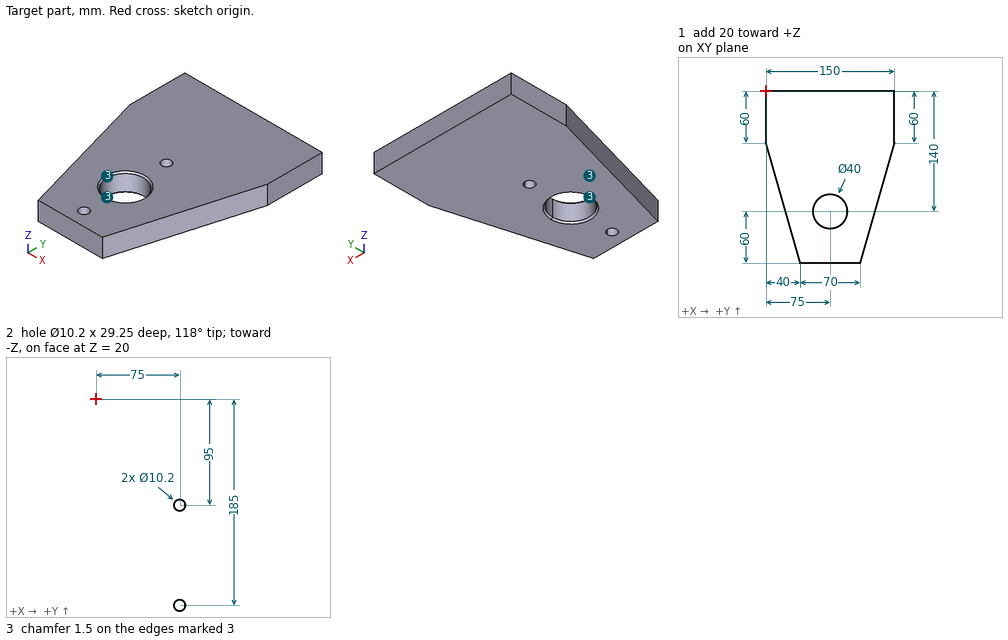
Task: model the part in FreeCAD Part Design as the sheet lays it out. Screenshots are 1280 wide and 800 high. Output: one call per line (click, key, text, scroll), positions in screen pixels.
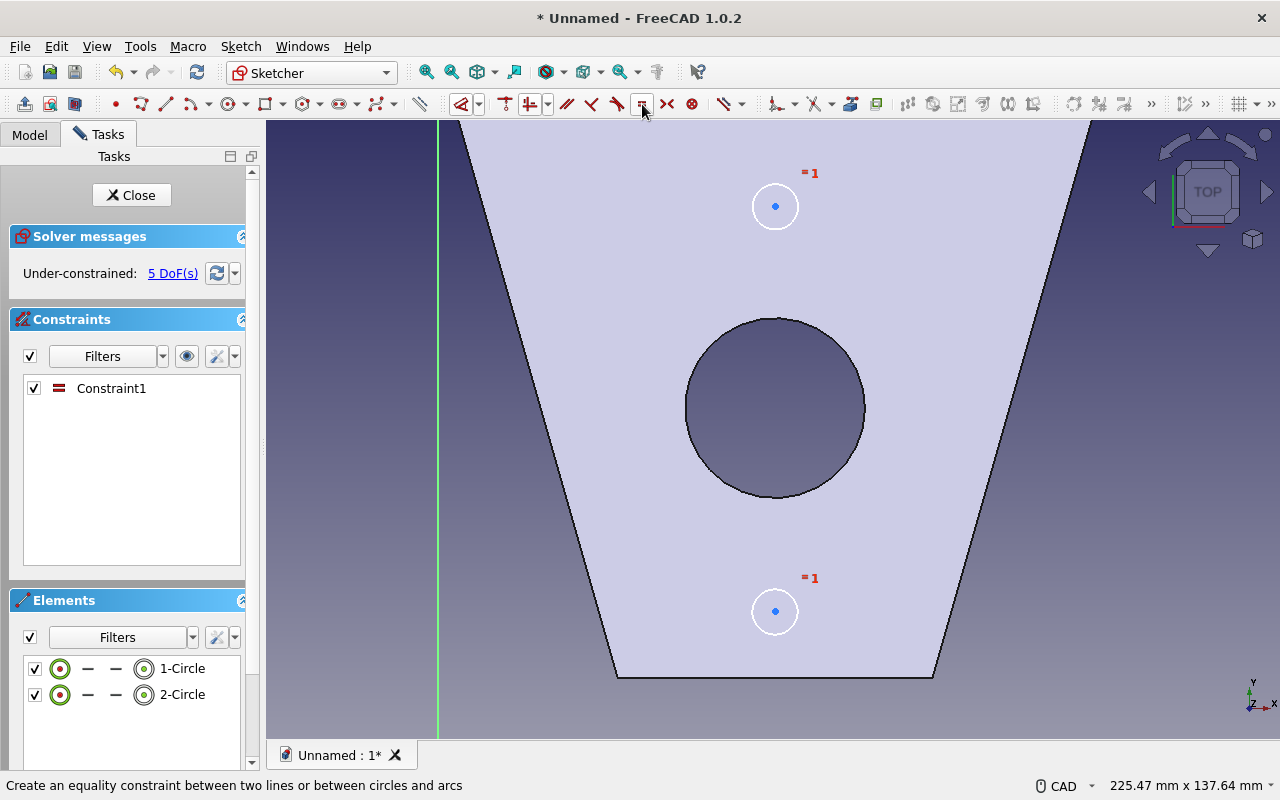
click(775, 207)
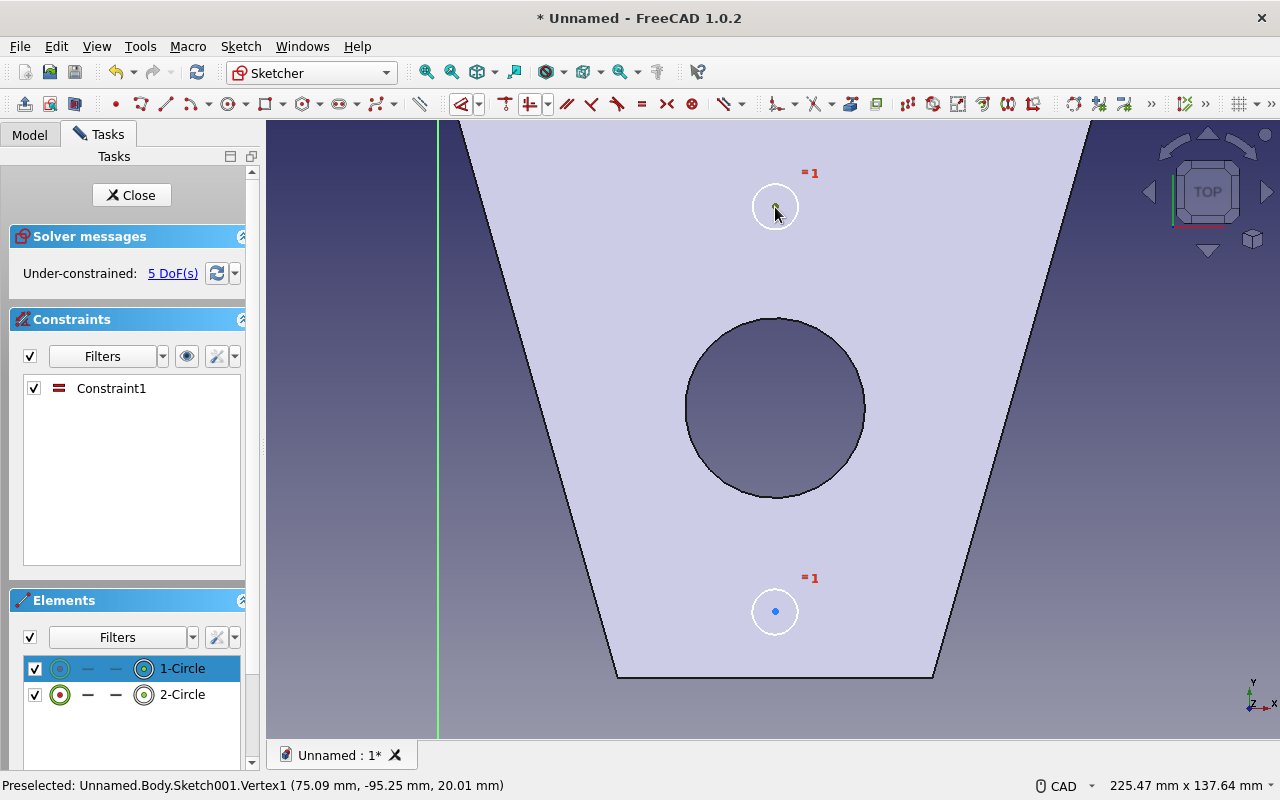
click(775, 612)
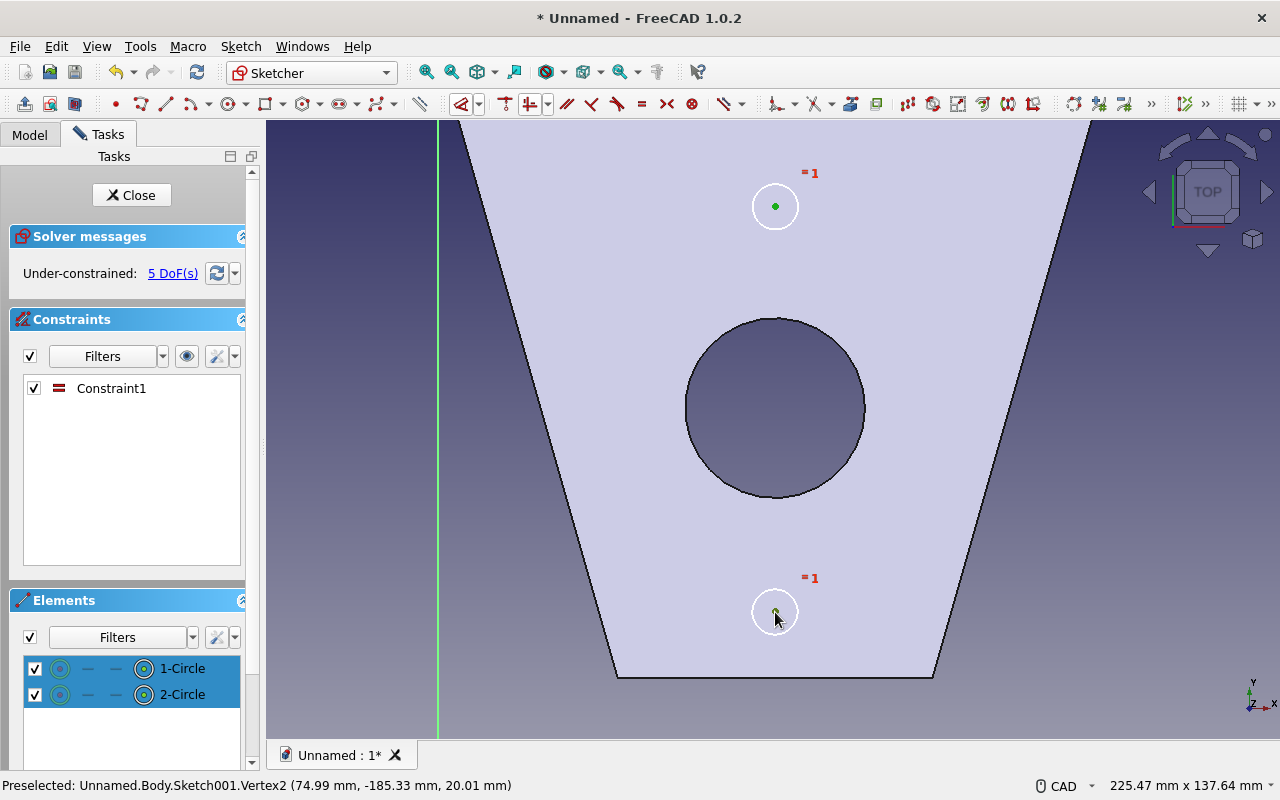
key(v)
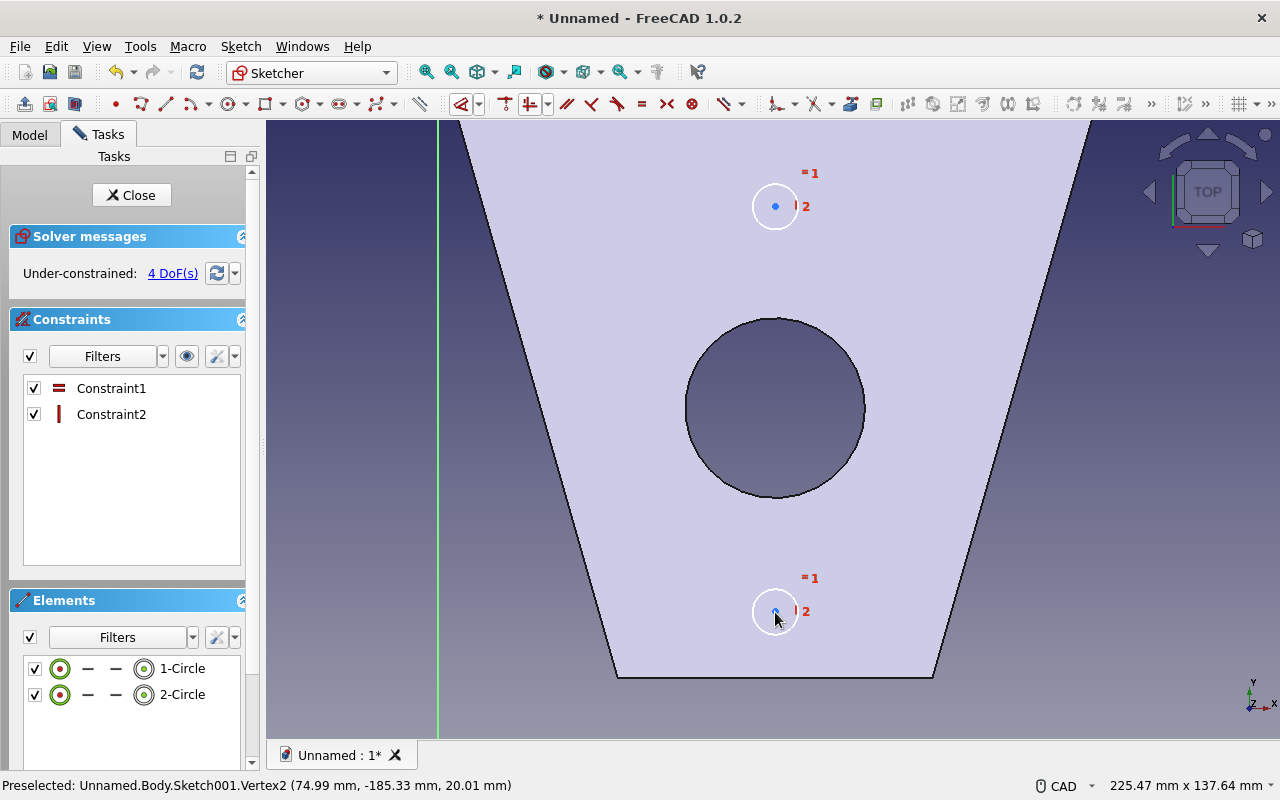
click(791, 191)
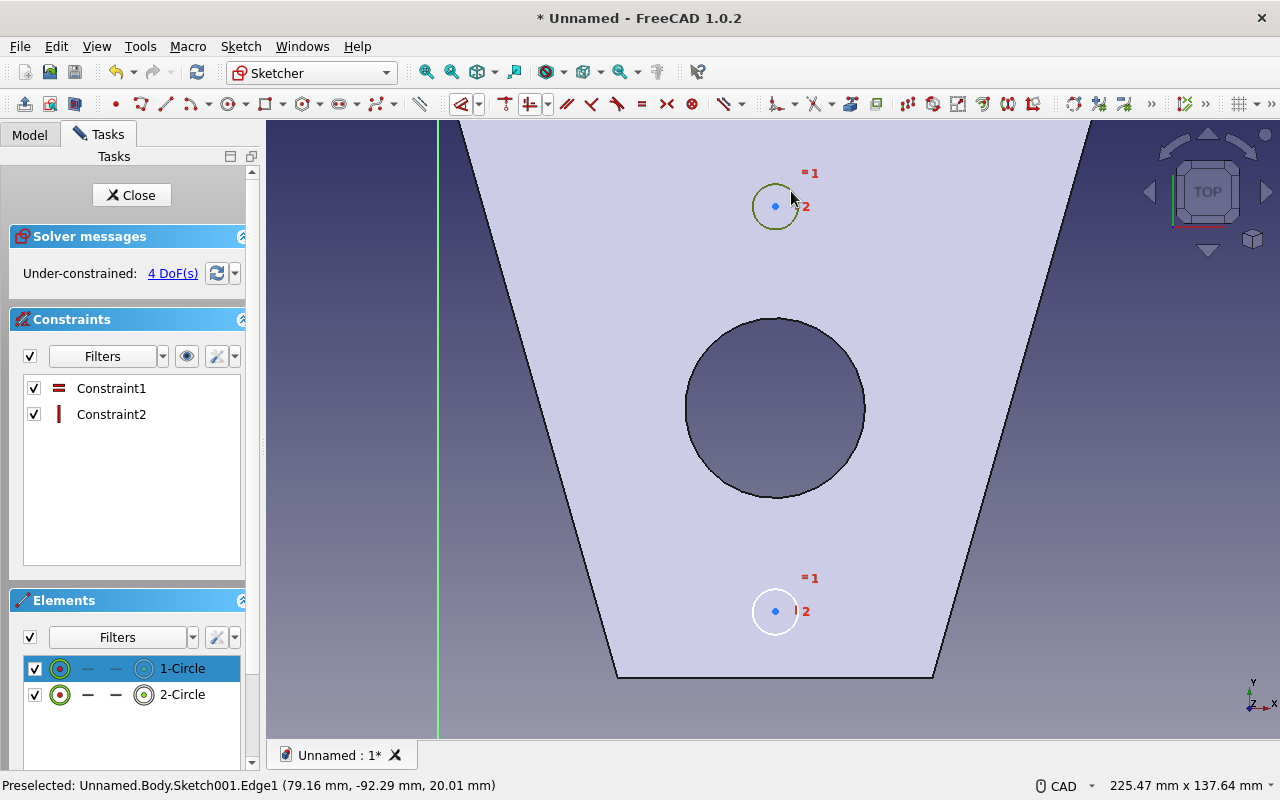
key(k)
key(o)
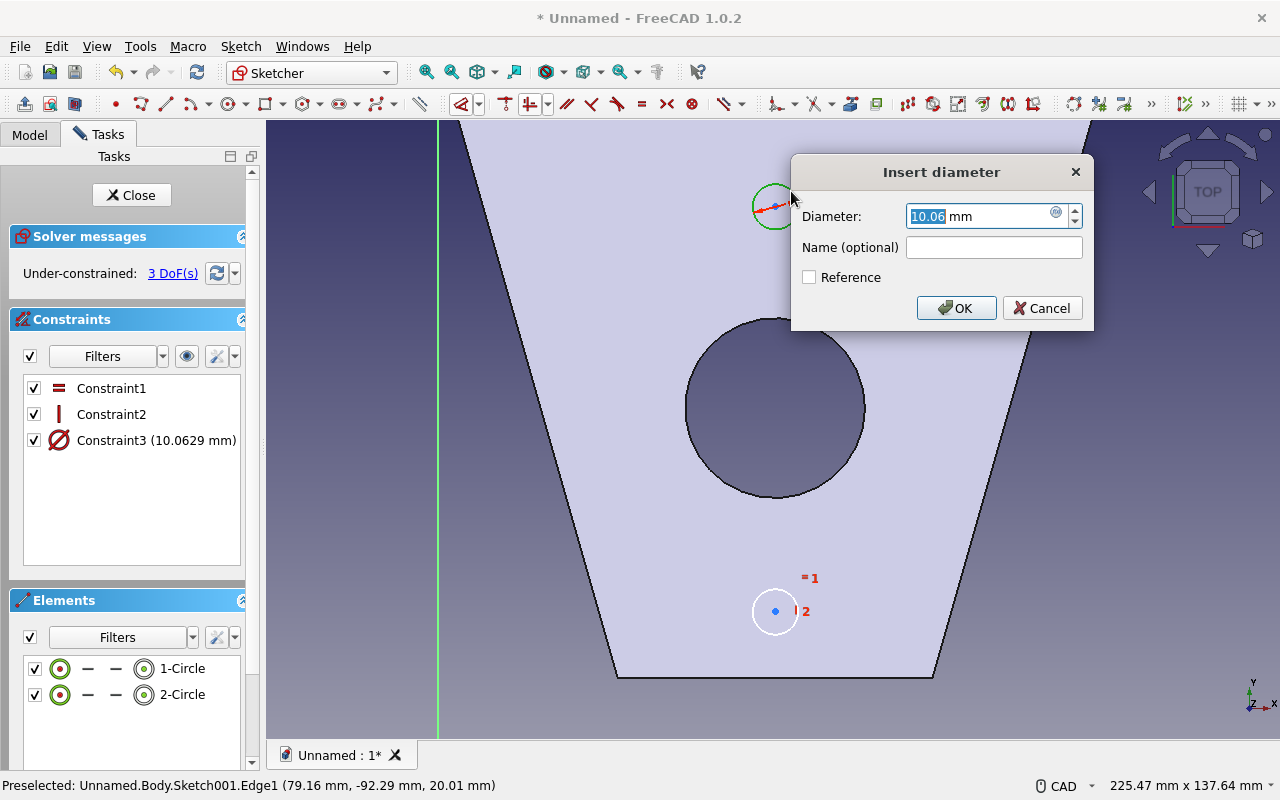
text(10.2)
key(Return)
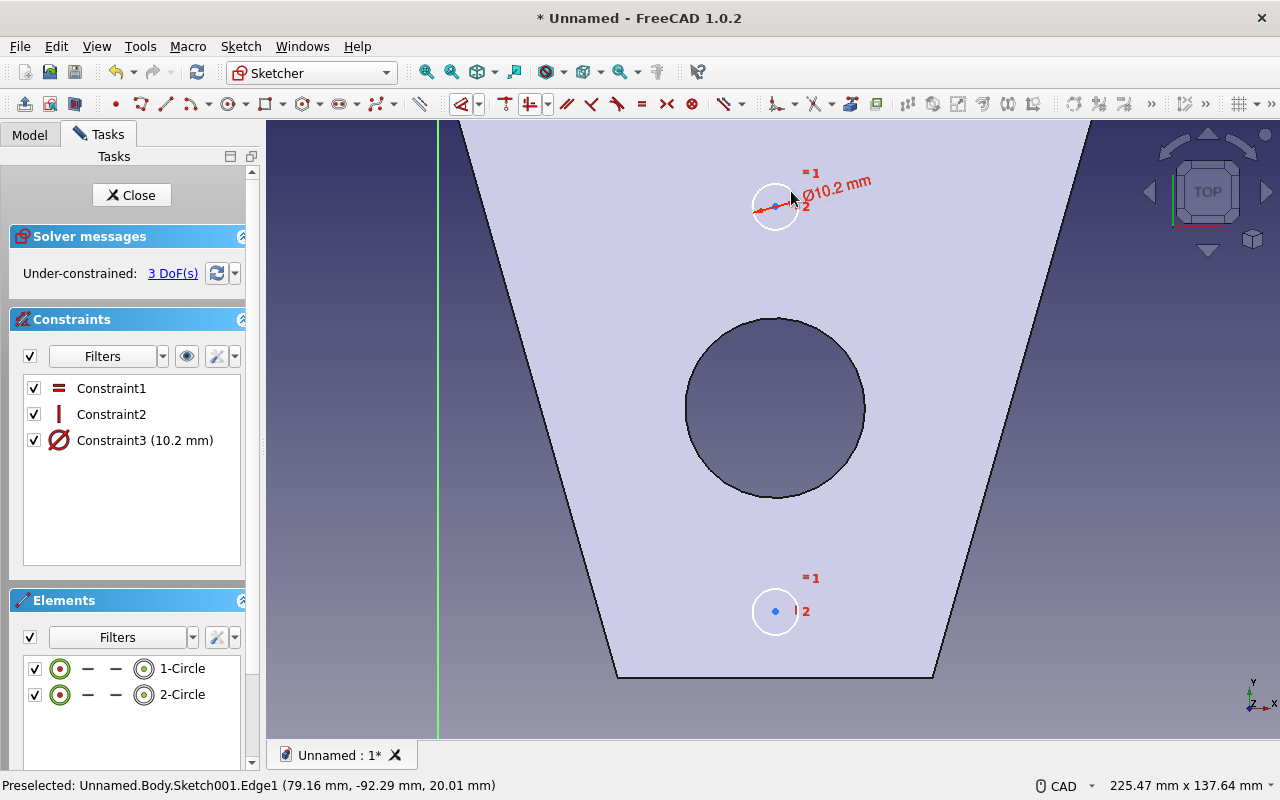
click(775, 207)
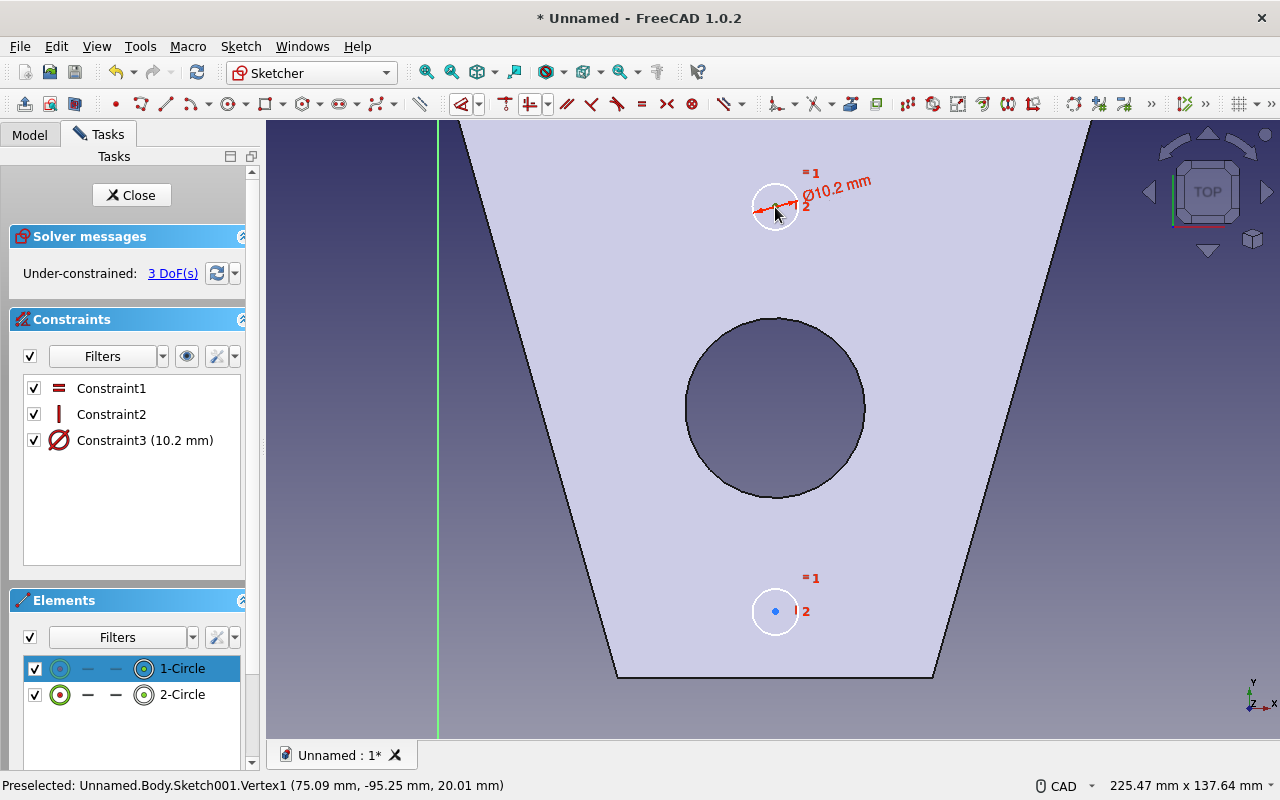
click(478, 104)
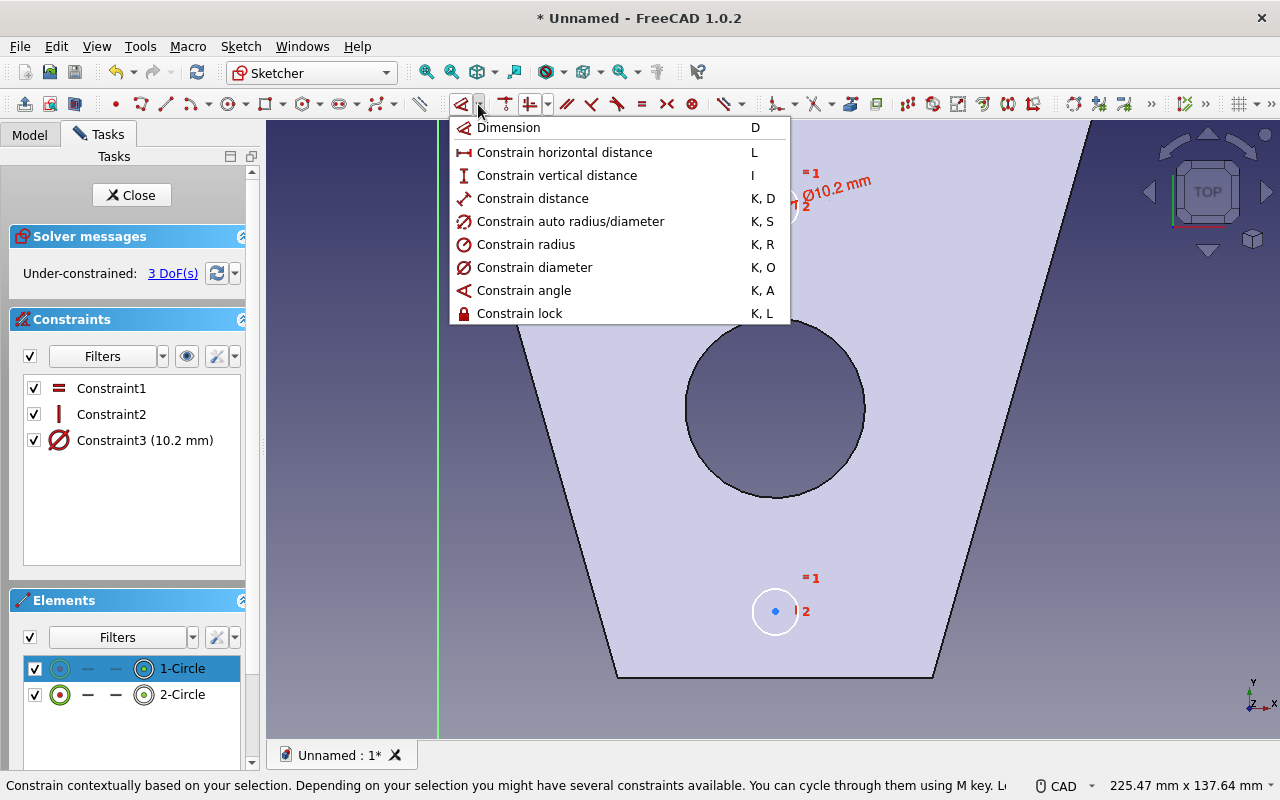
click(620, 152)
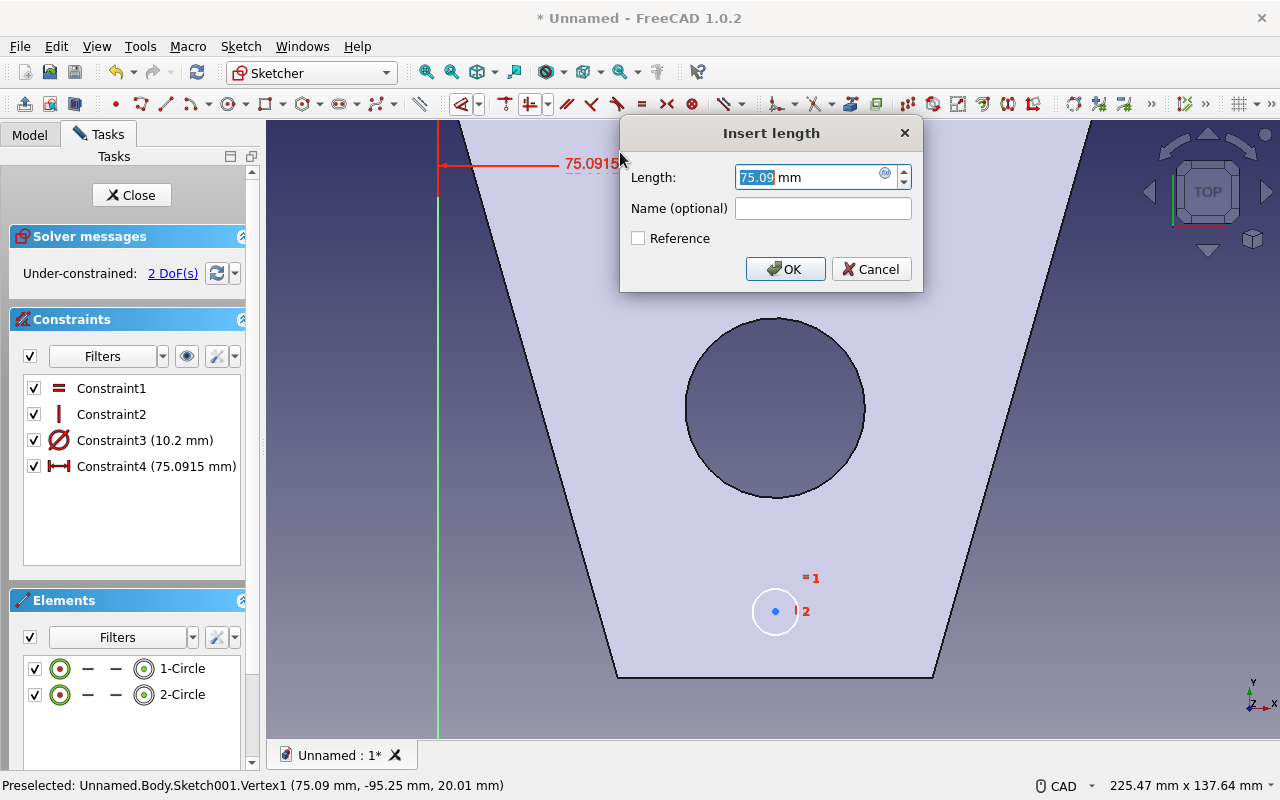
text(75)
key(Return)